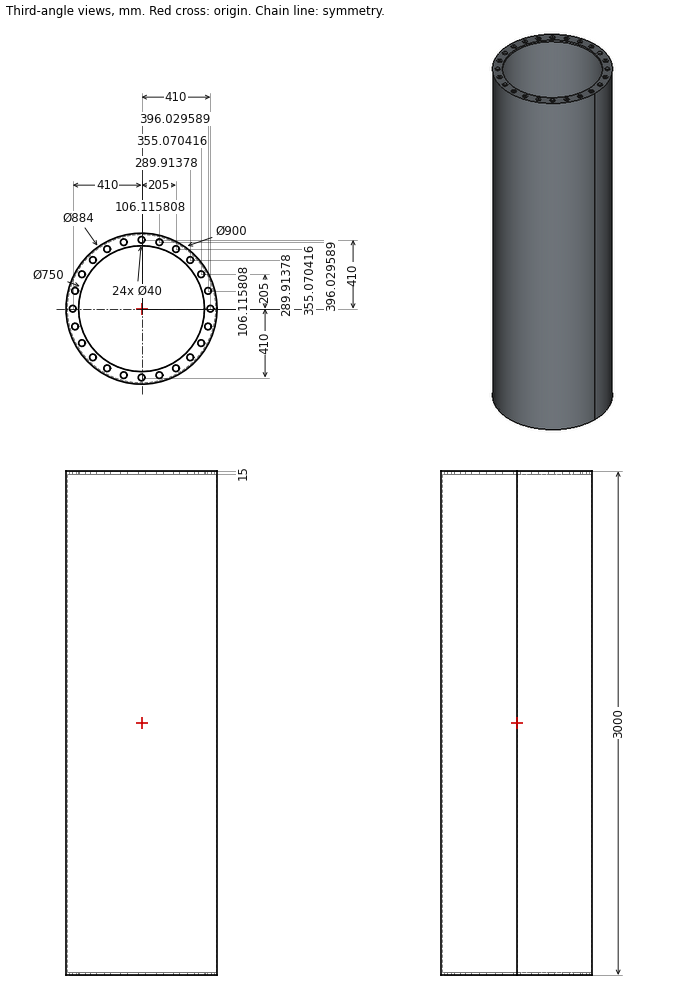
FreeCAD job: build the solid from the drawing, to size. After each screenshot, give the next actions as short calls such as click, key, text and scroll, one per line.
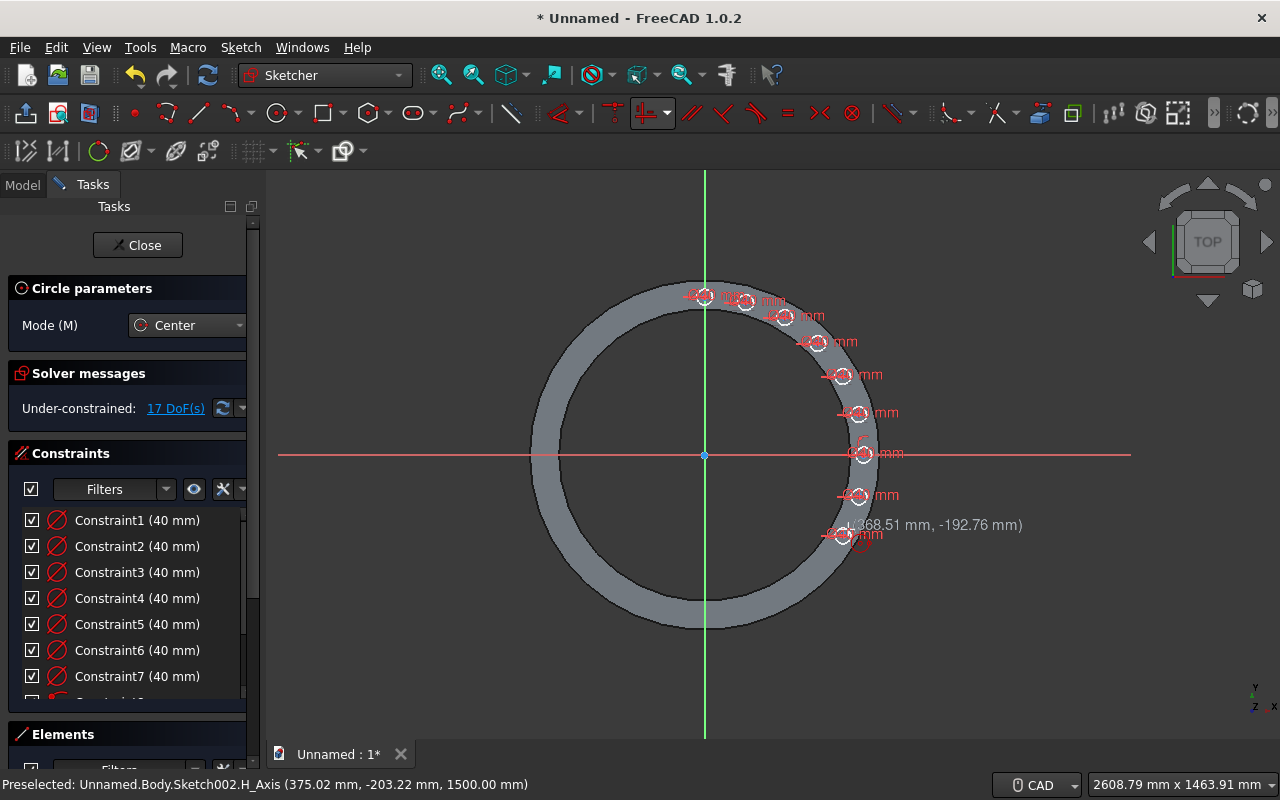
scroll(817, 568, up, 6)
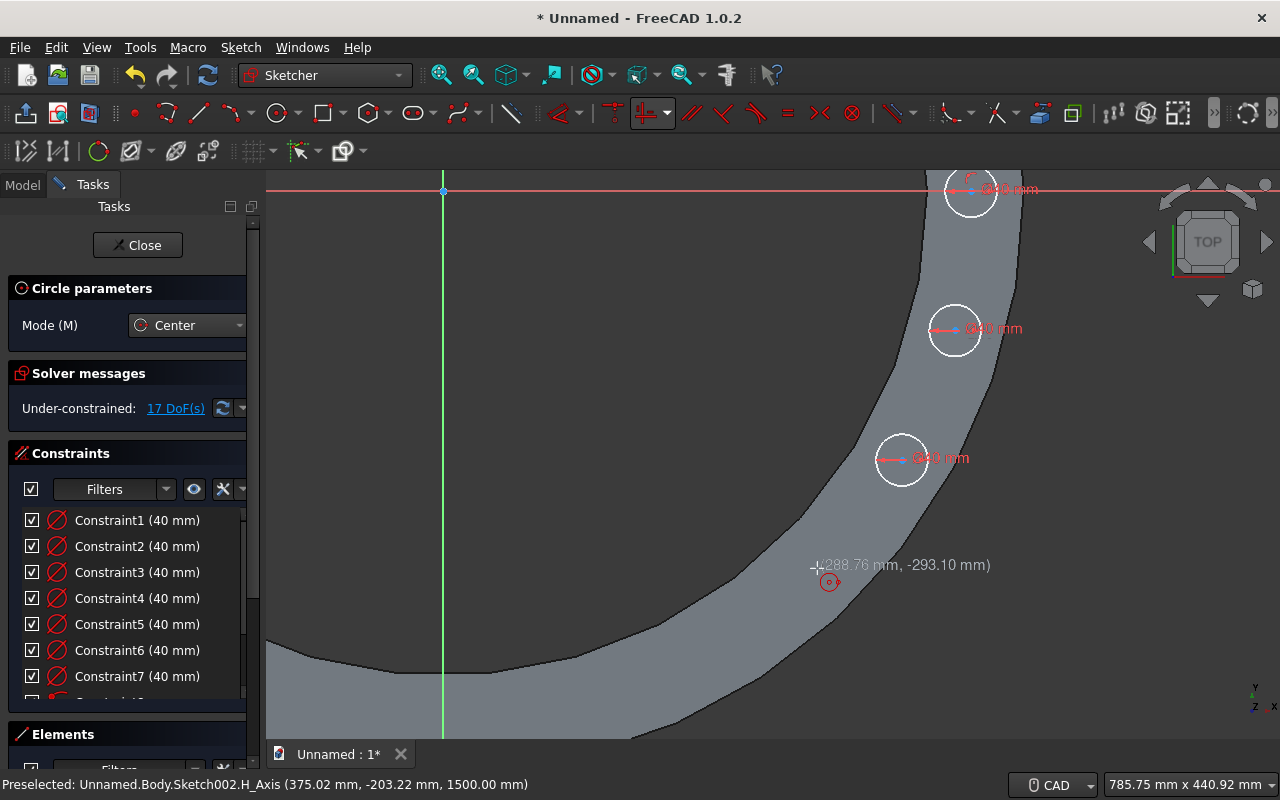
scroll(817, 568, down, 6)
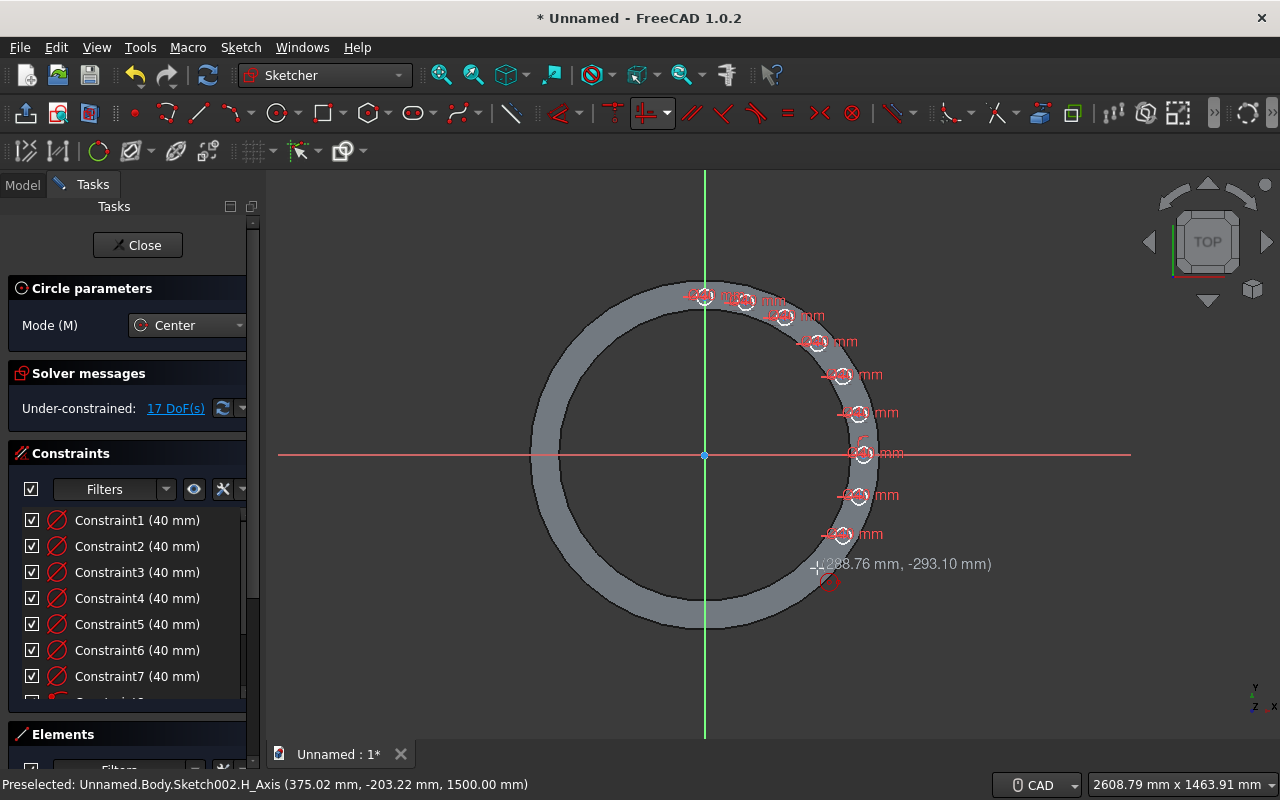
click(817, 568)
move(823, 562)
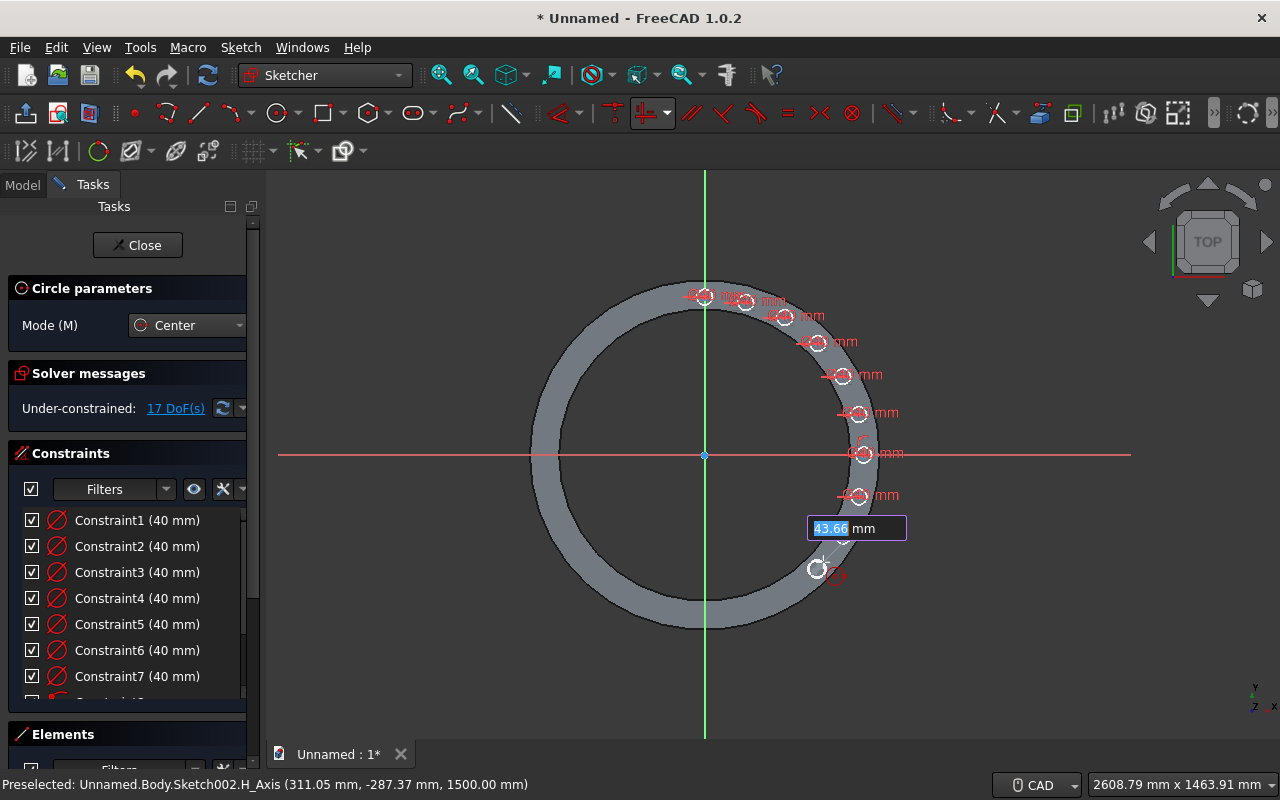
text(40)
key(Return)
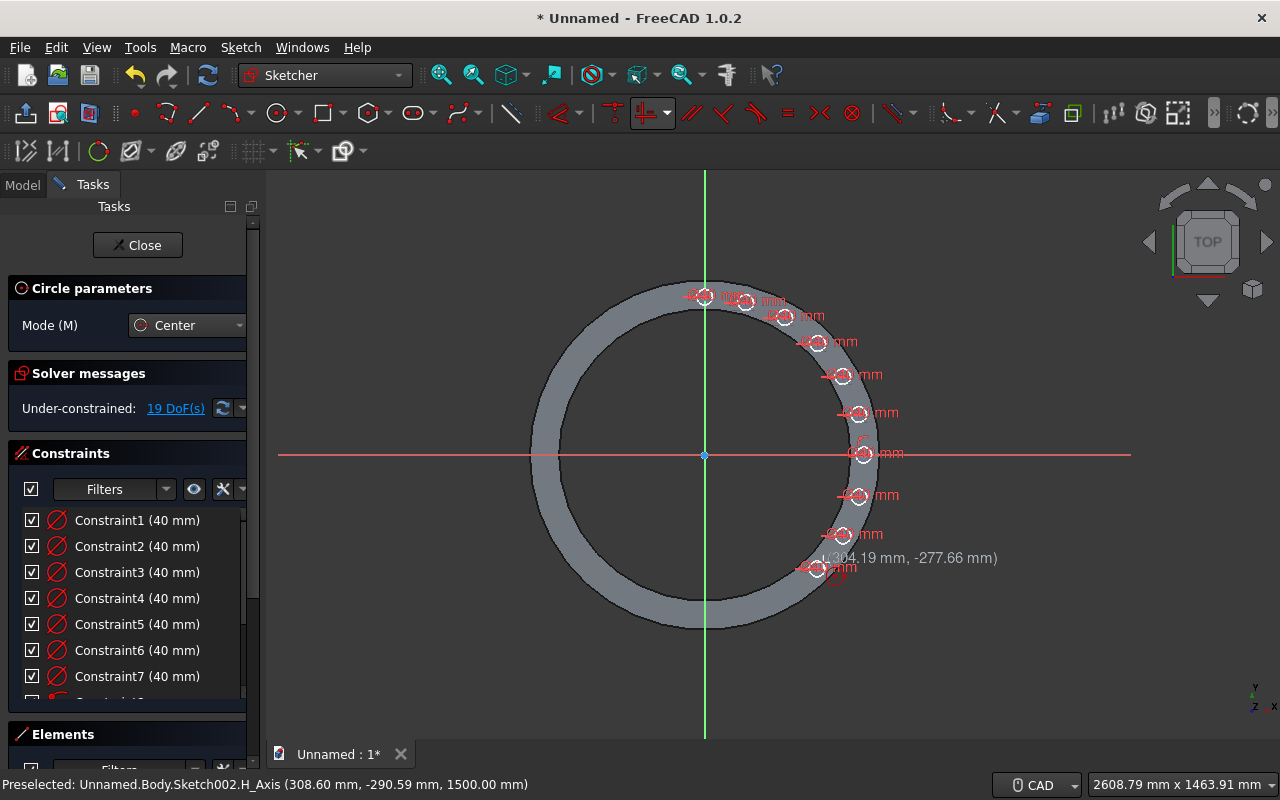
scroll(784, 593, up, 6)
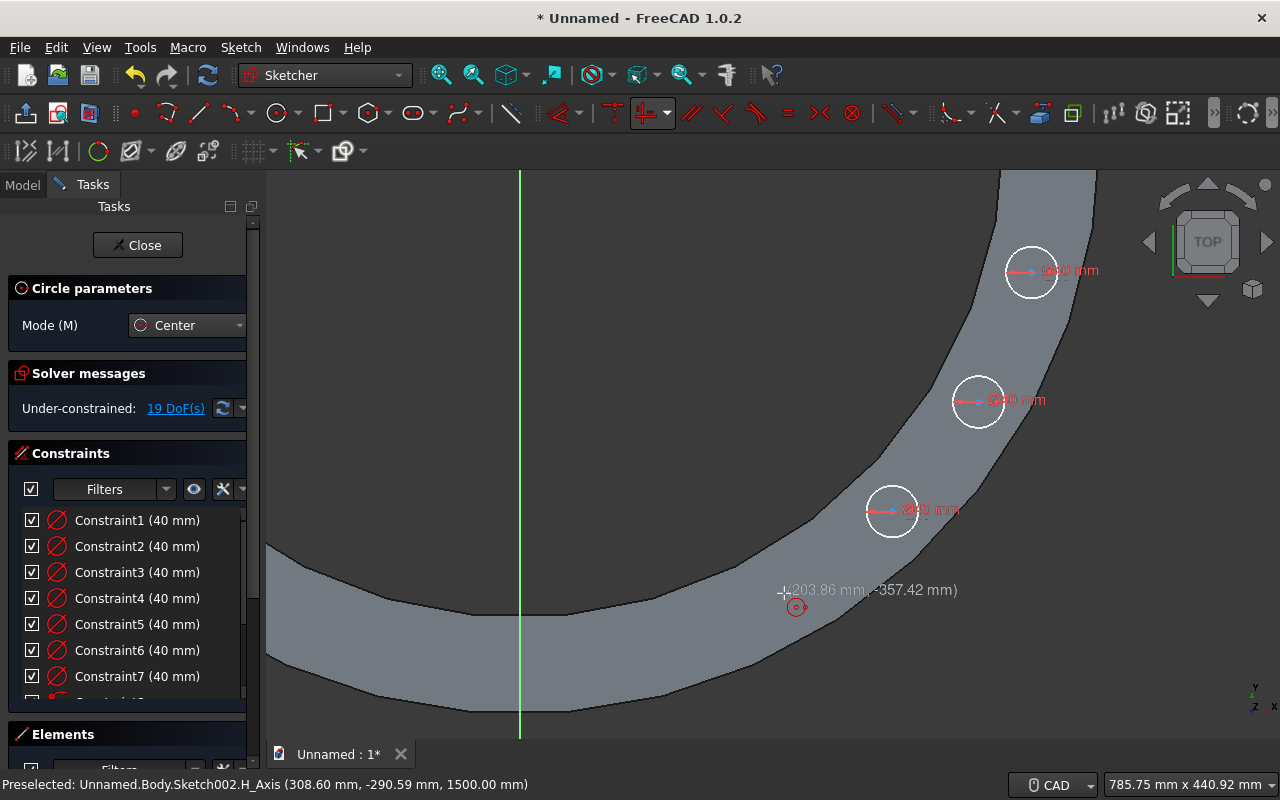
scroll(784, 593, down, 6)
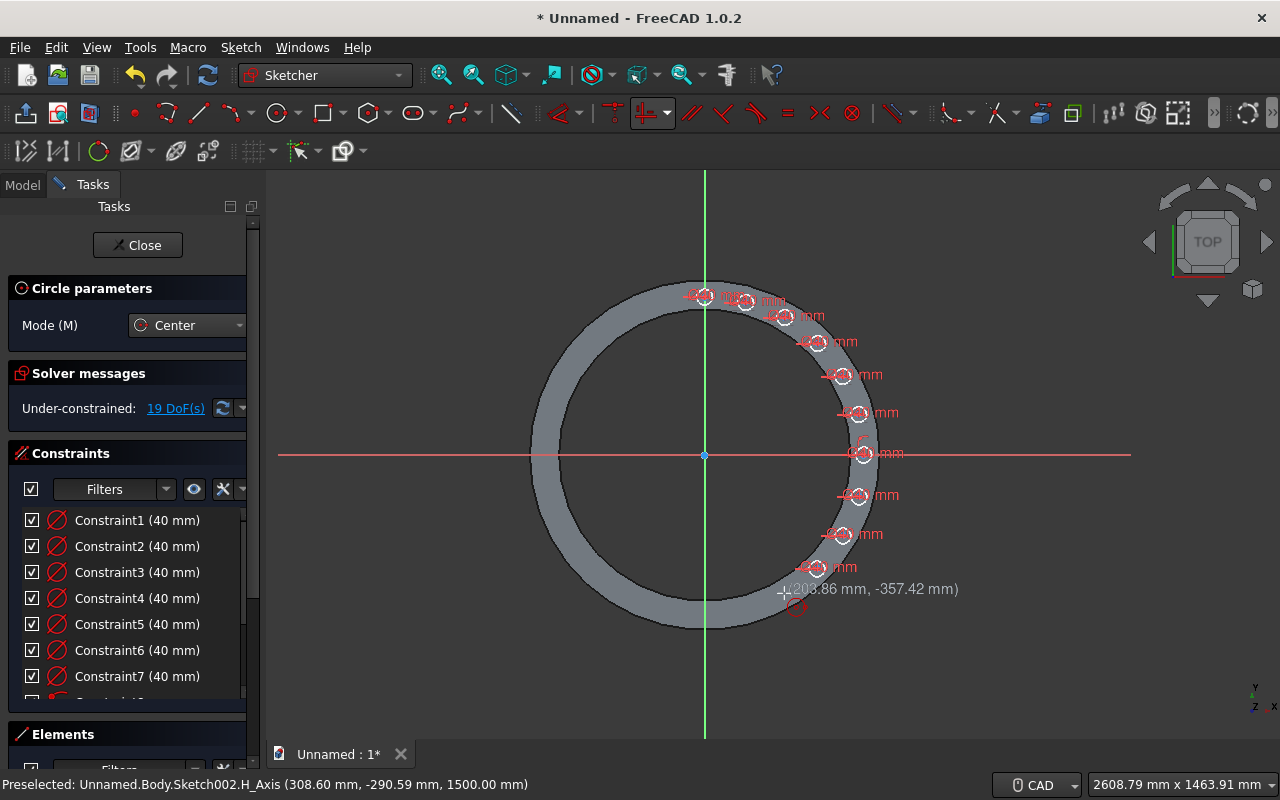
click(784, 593)
move(790, 588)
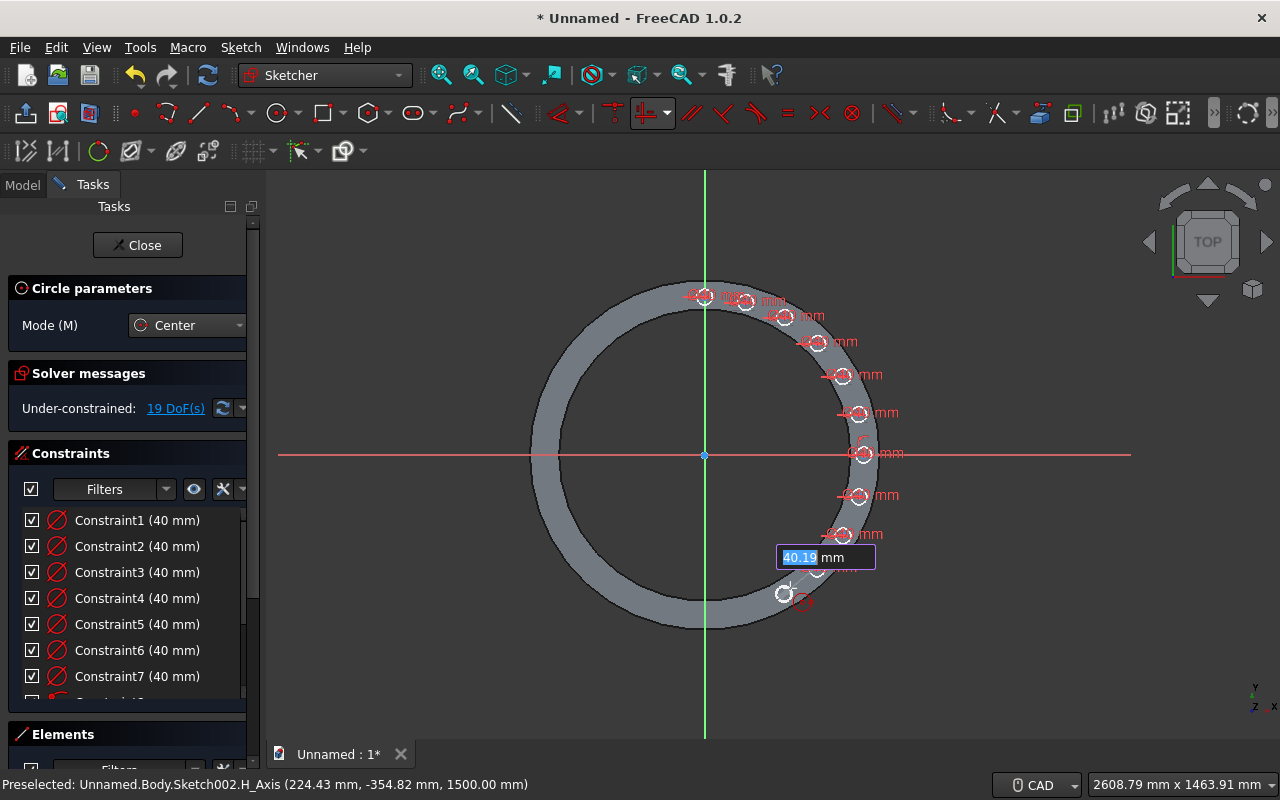
text(40)
key(Return)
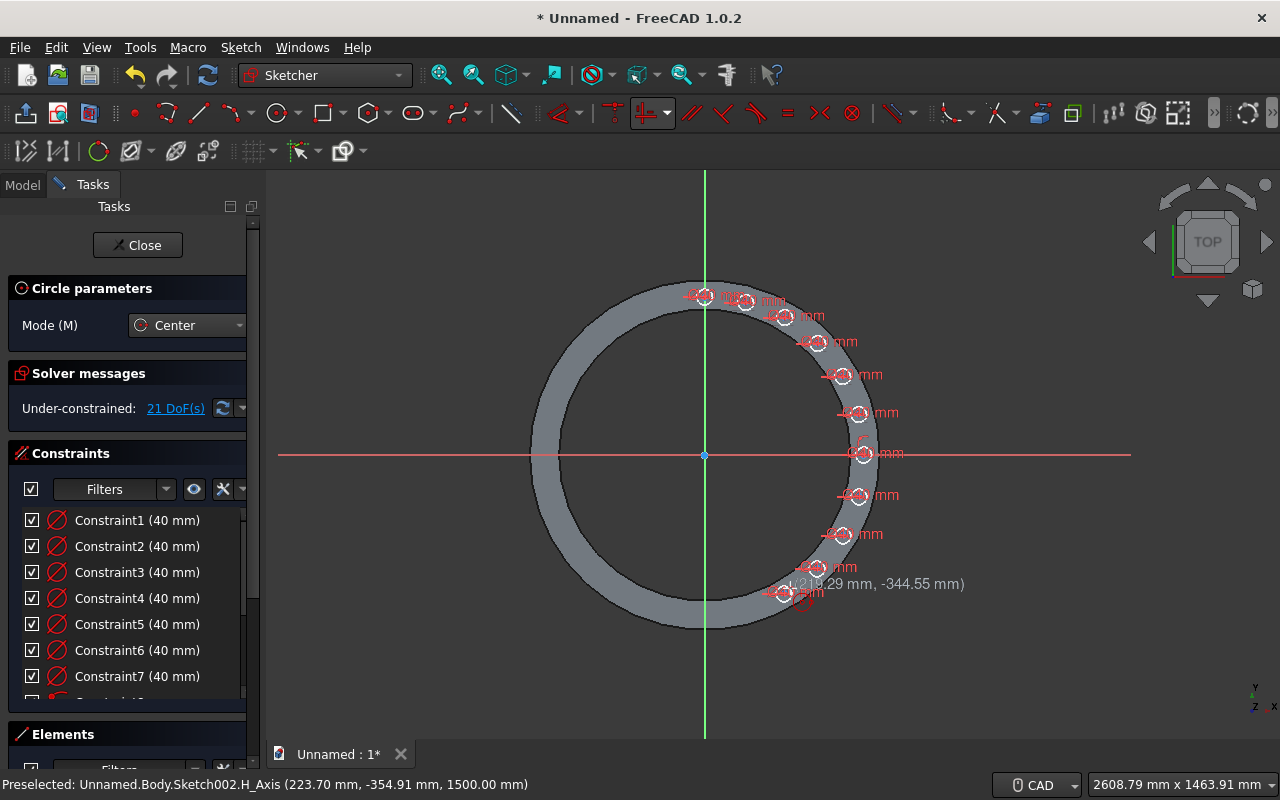
scroll(746, 609, up, 6)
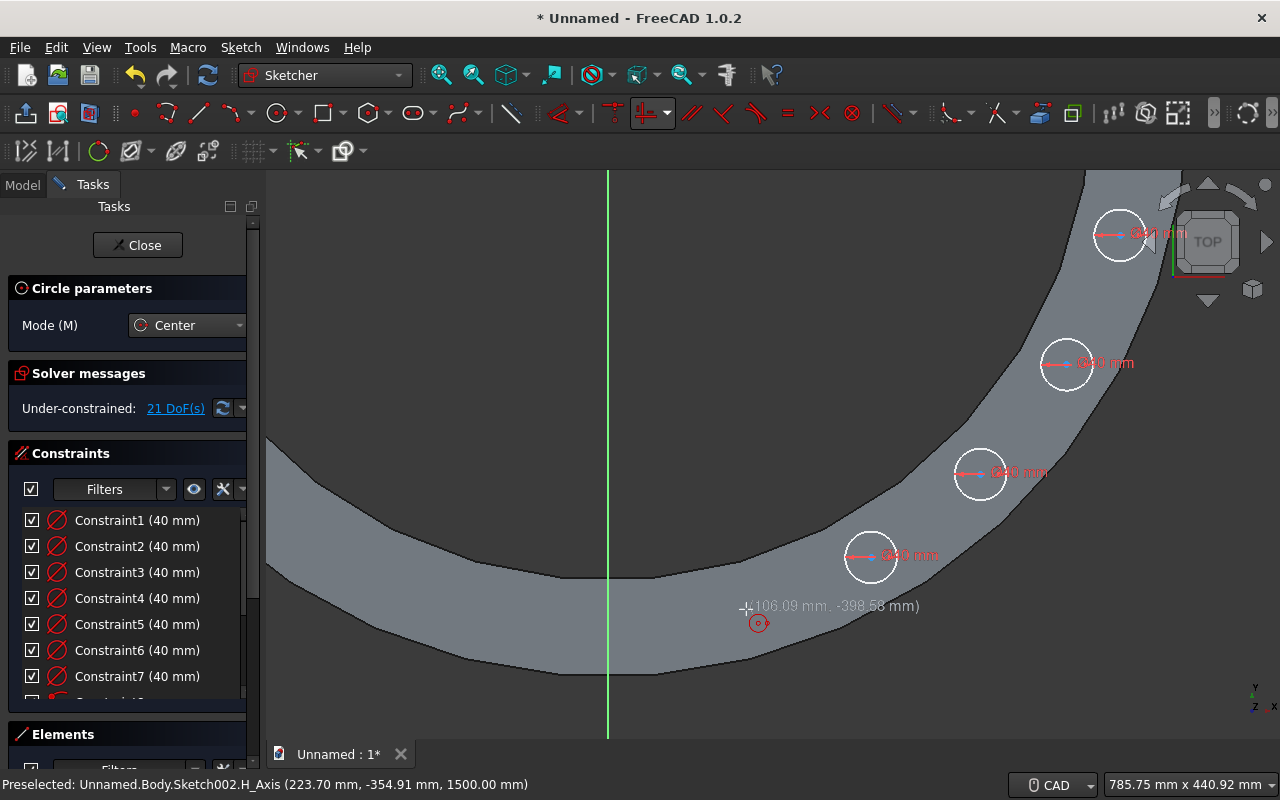
scroll(746, 609, down, 6)